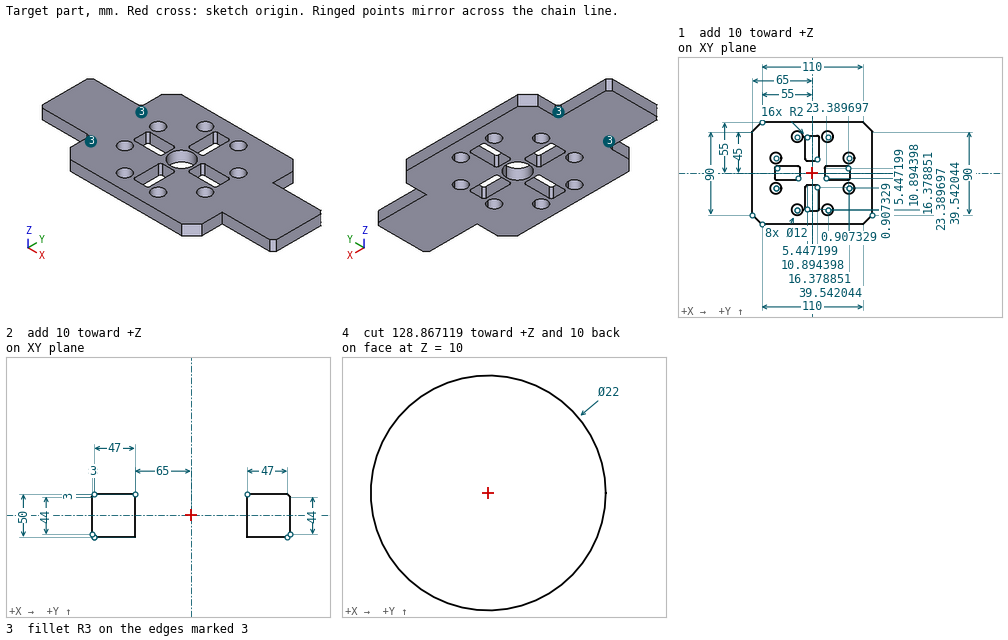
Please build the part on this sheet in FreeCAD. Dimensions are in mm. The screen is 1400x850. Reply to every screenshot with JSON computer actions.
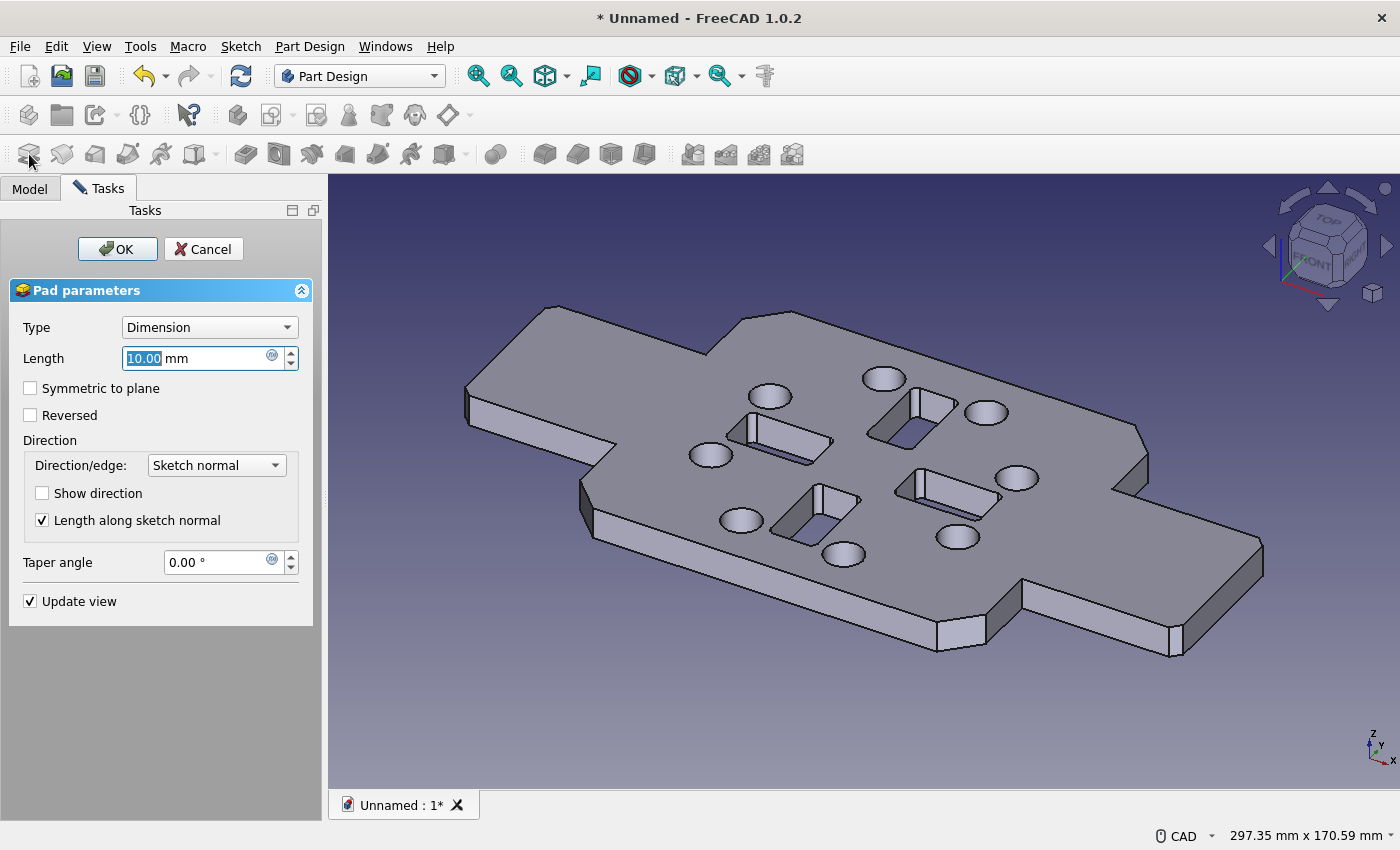
{"action": "type", "text": "10"}
{"action": "key", "text": "Tab"}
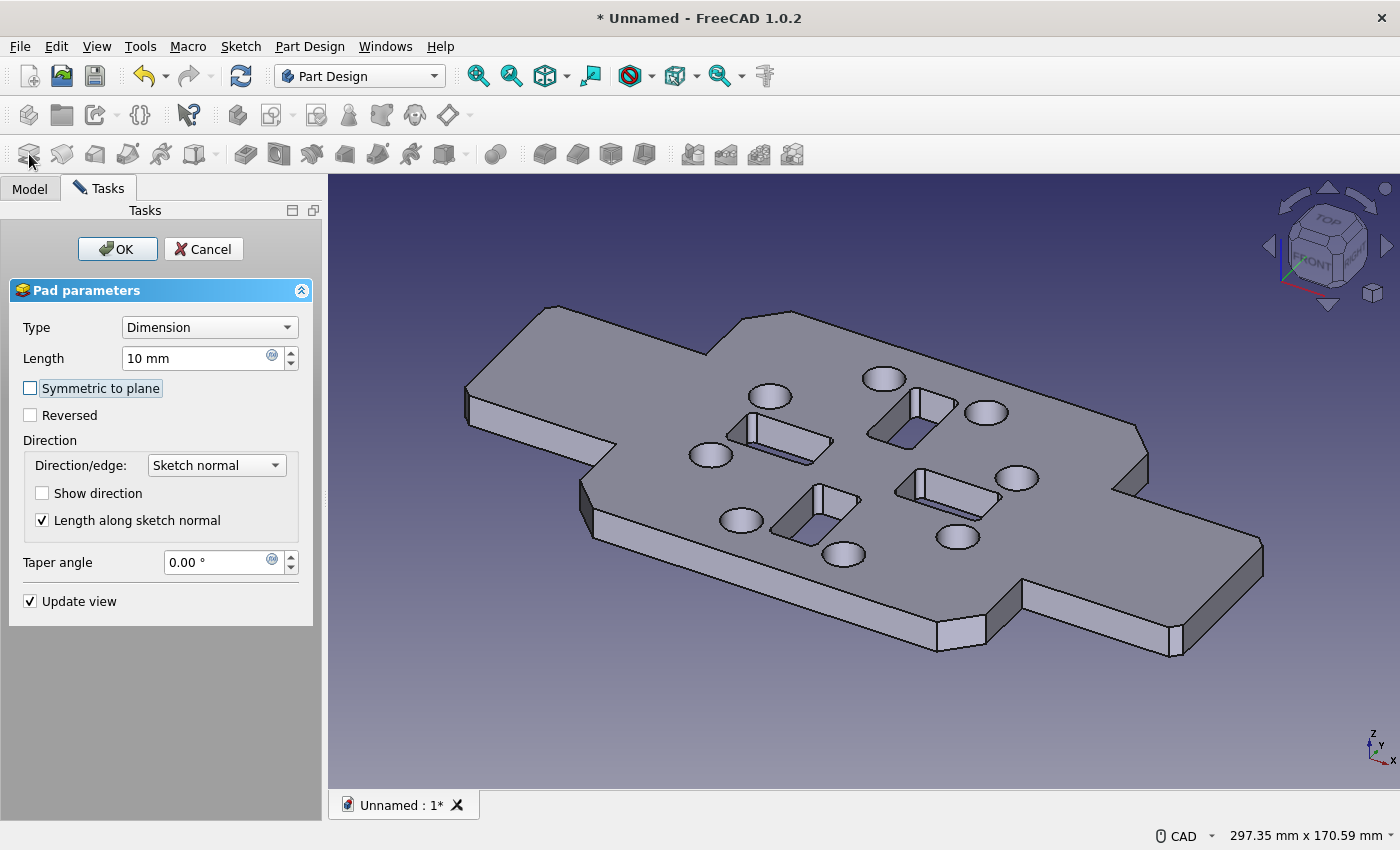
{"action": "left_click", "coordinate": [118, 249]}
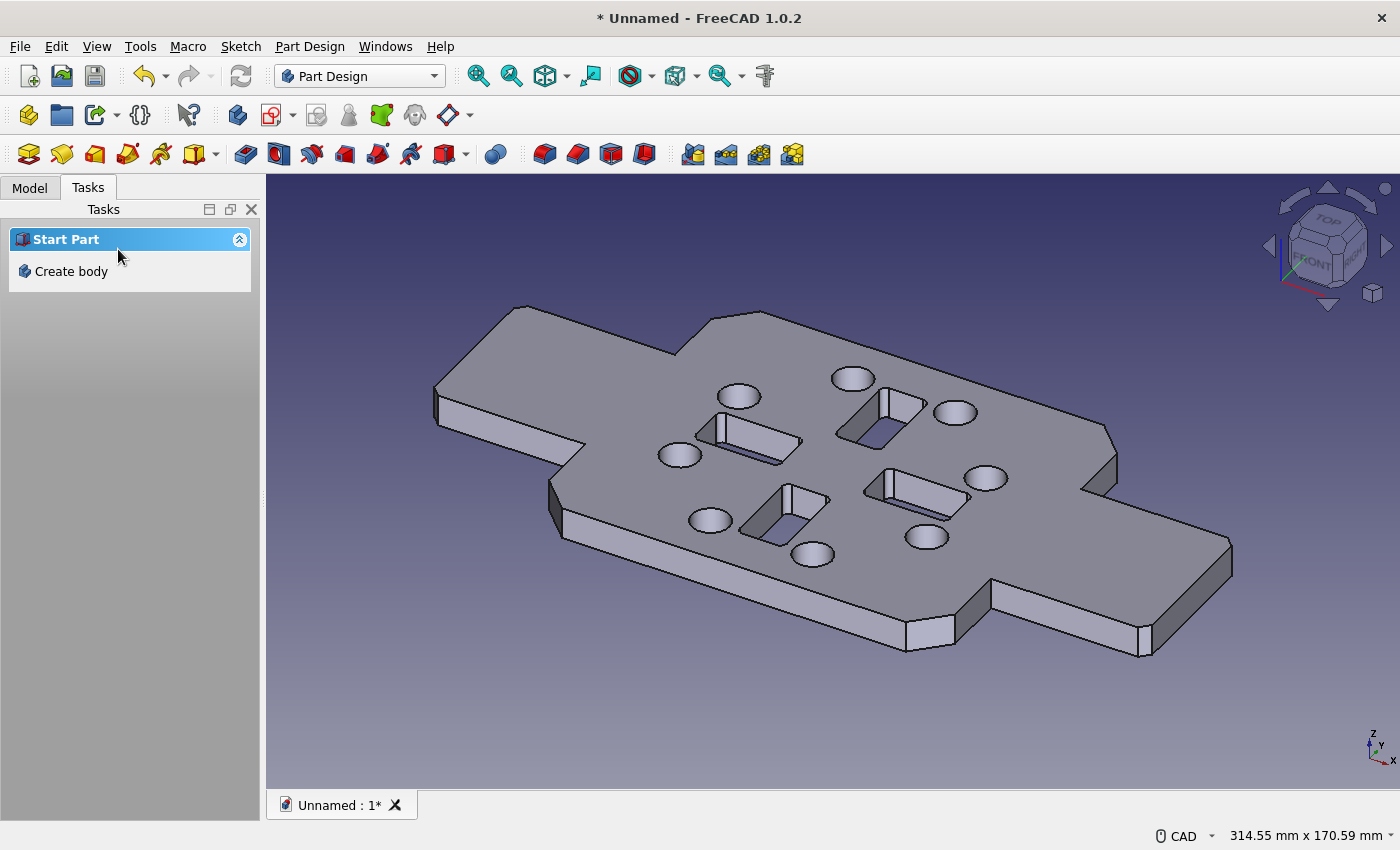
{"action": "key", "text": "0"}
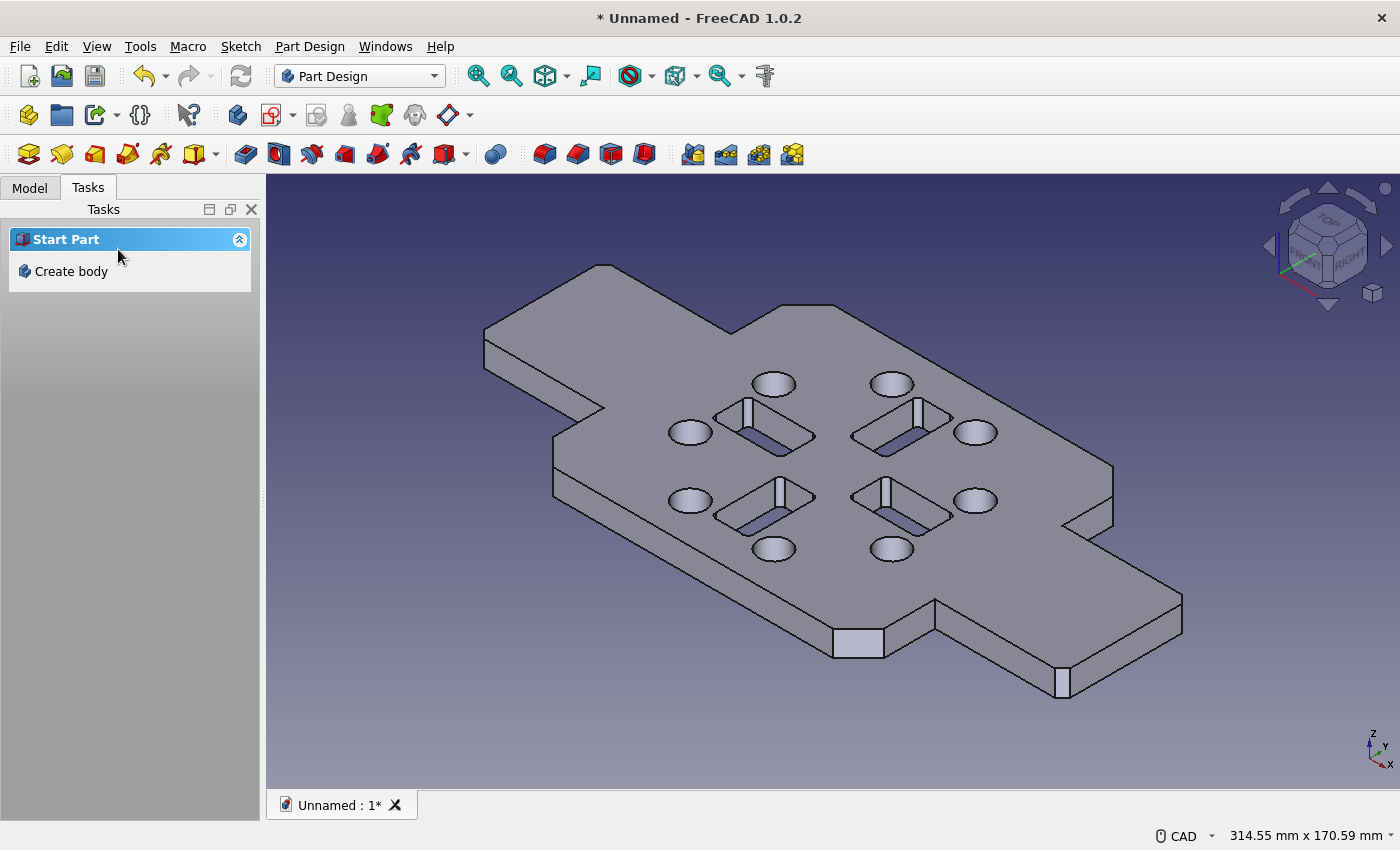
{"action": "key", "text": "2"}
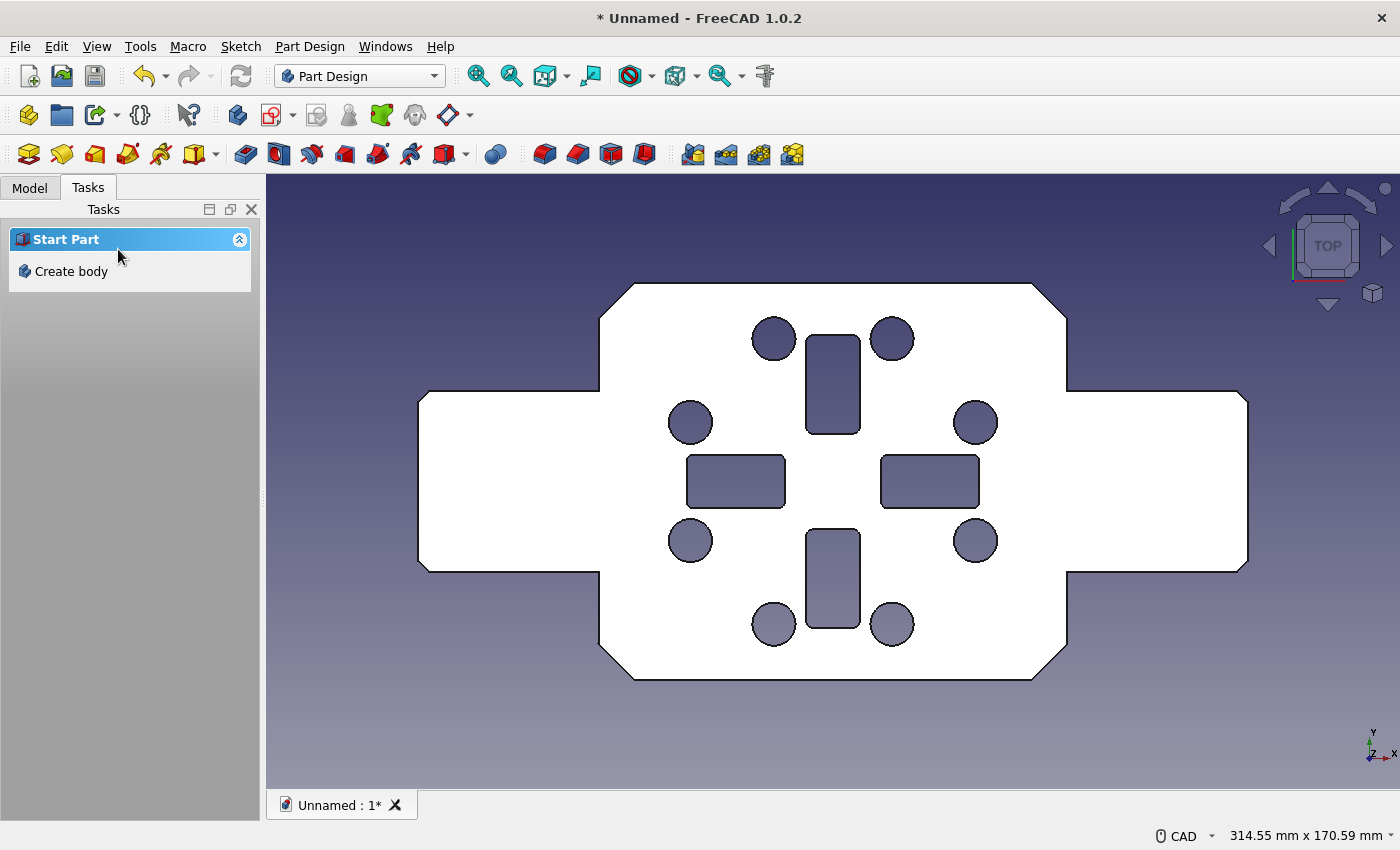
{"action": "key", "text": "1"}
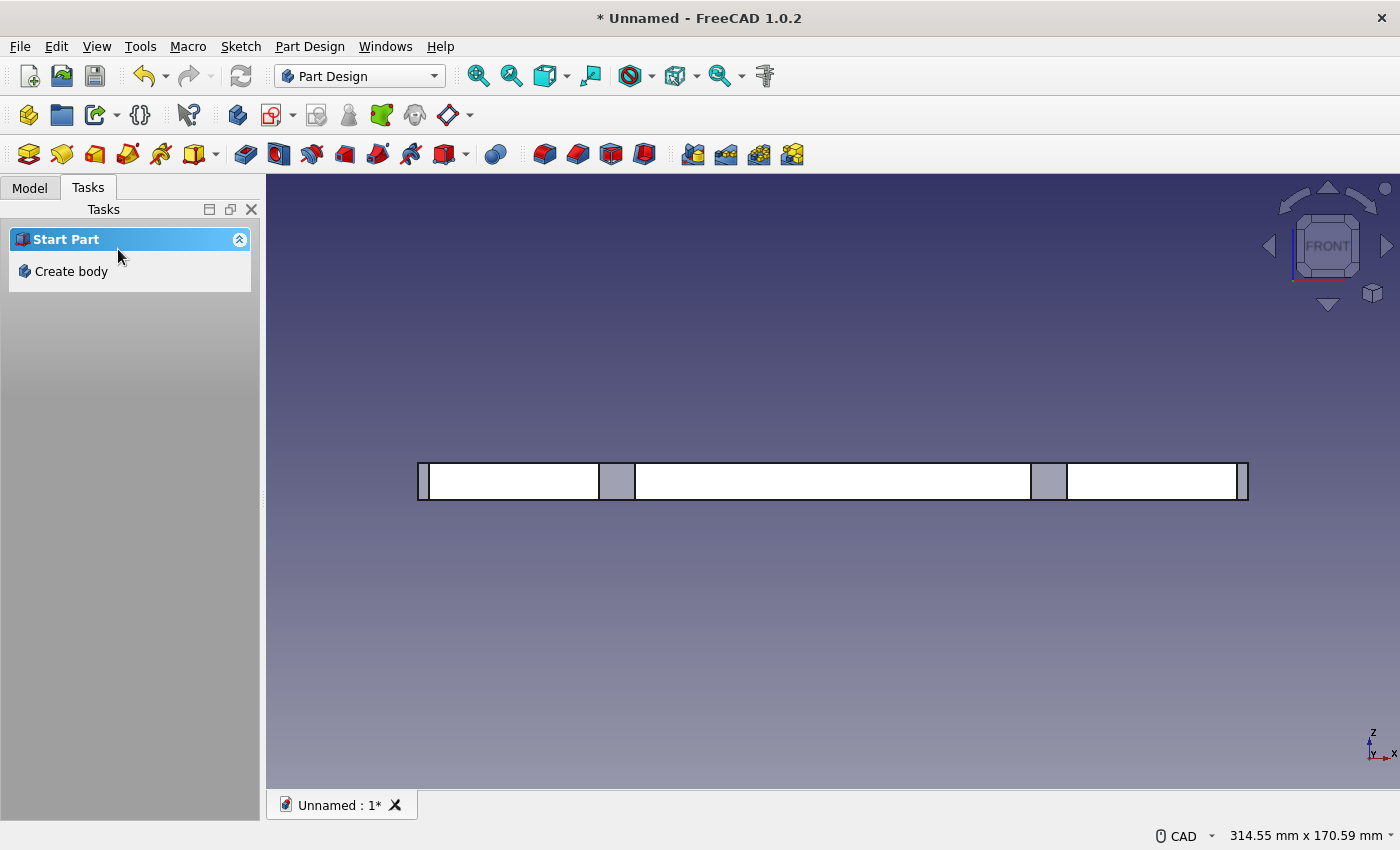
{"action": "key", "text": "3"}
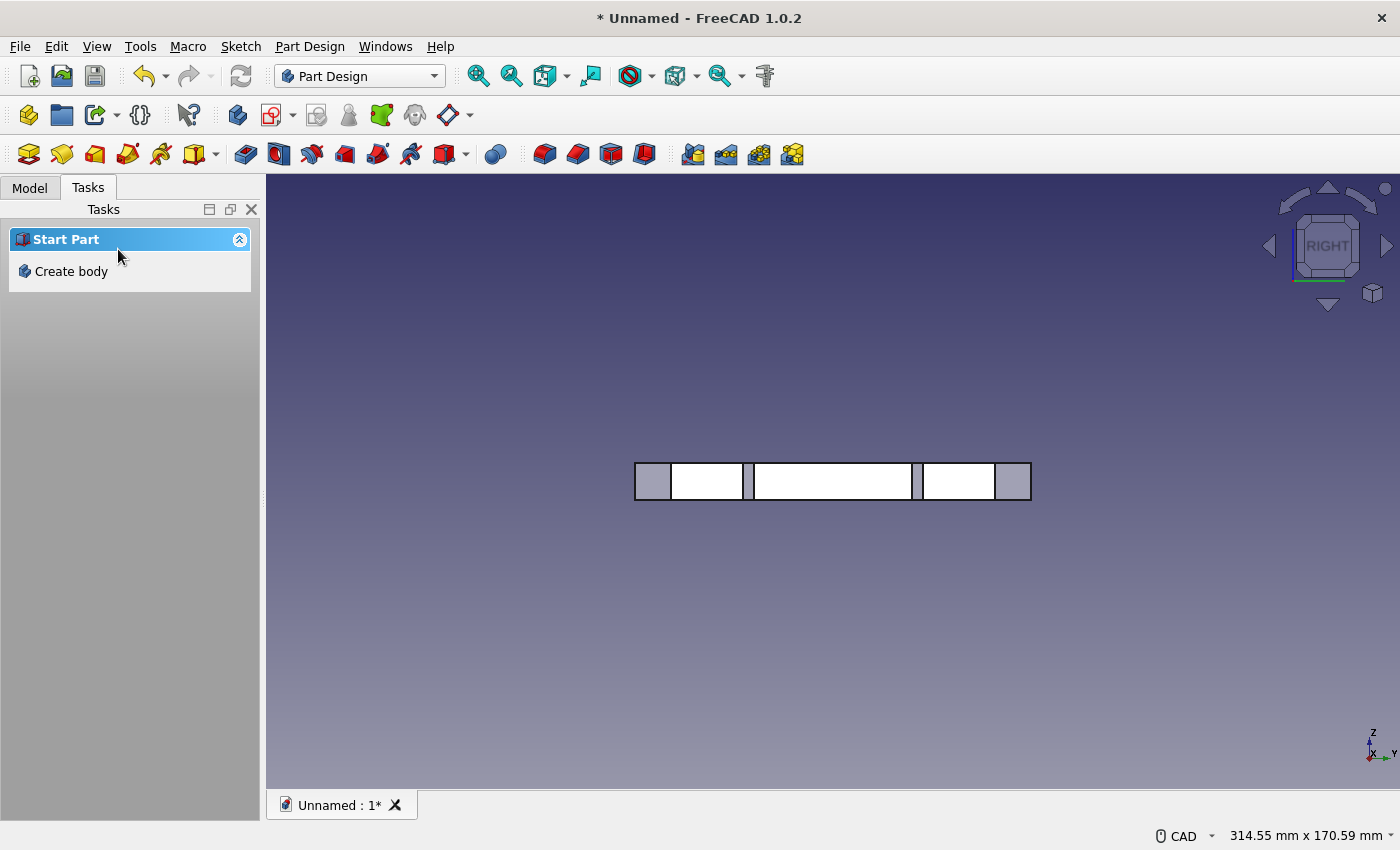
{"action": "left_click", "coordinate": [479, 76]}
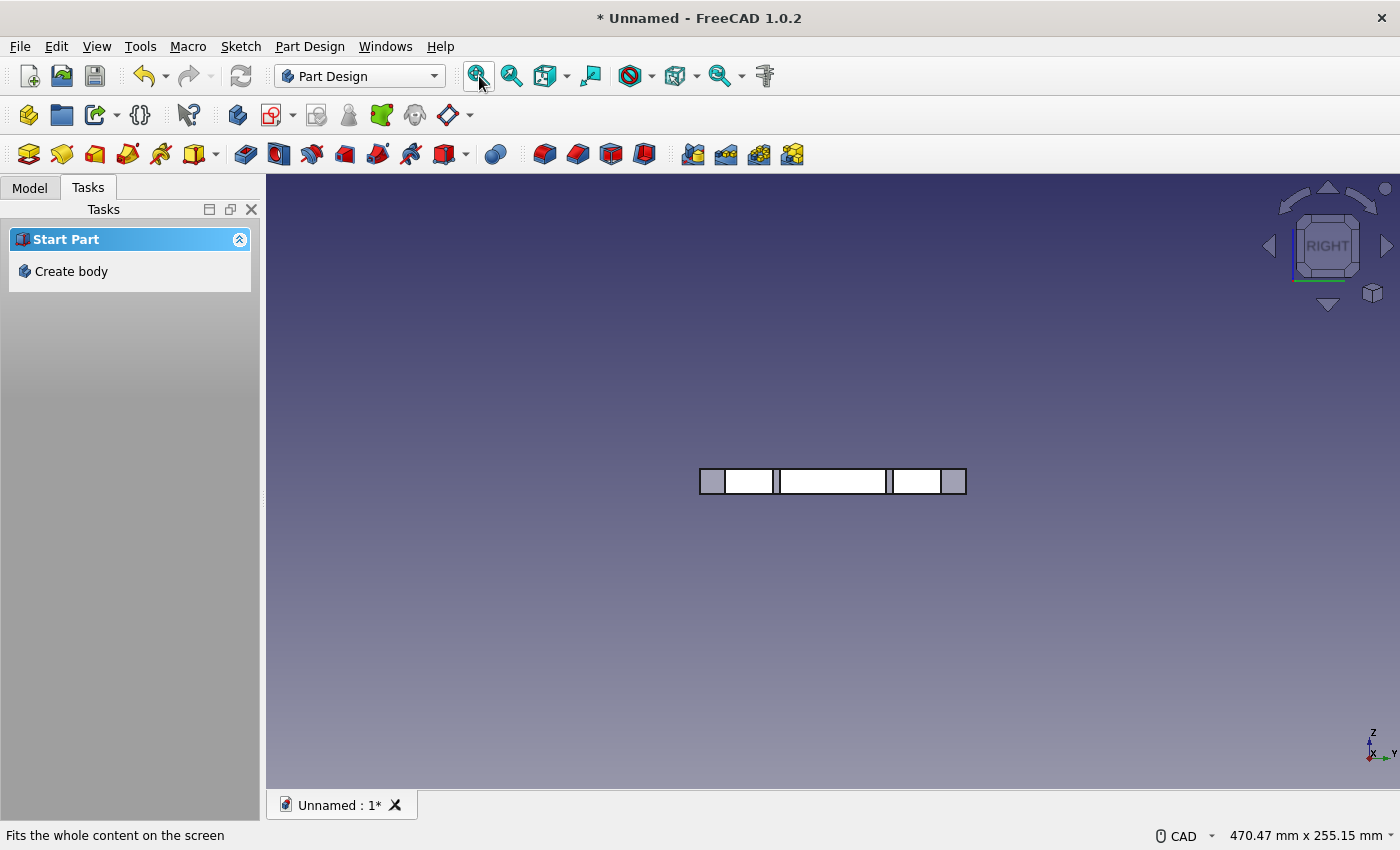
{"action": "key", "text": "5"}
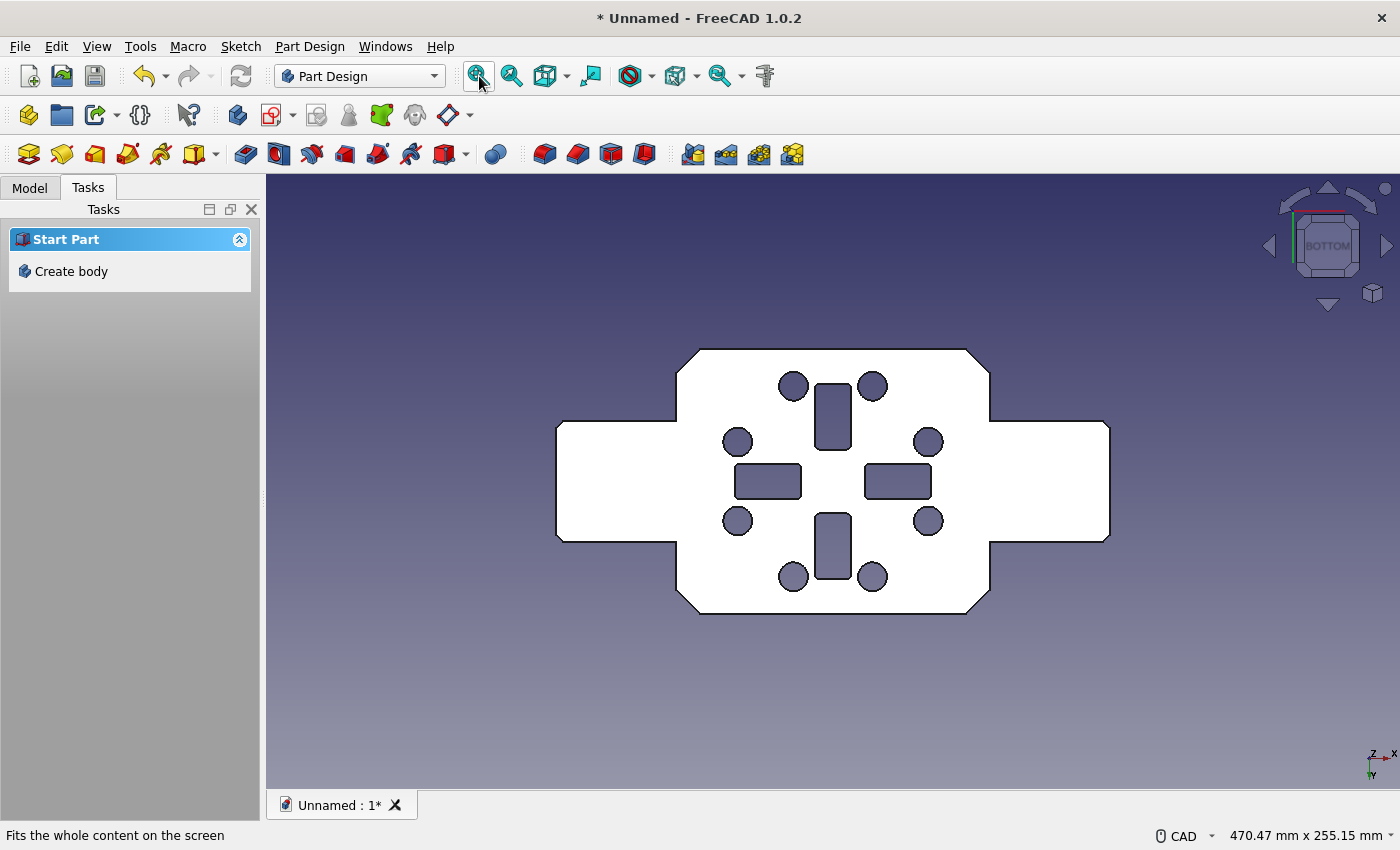
{"action": "key", "text": "4"}